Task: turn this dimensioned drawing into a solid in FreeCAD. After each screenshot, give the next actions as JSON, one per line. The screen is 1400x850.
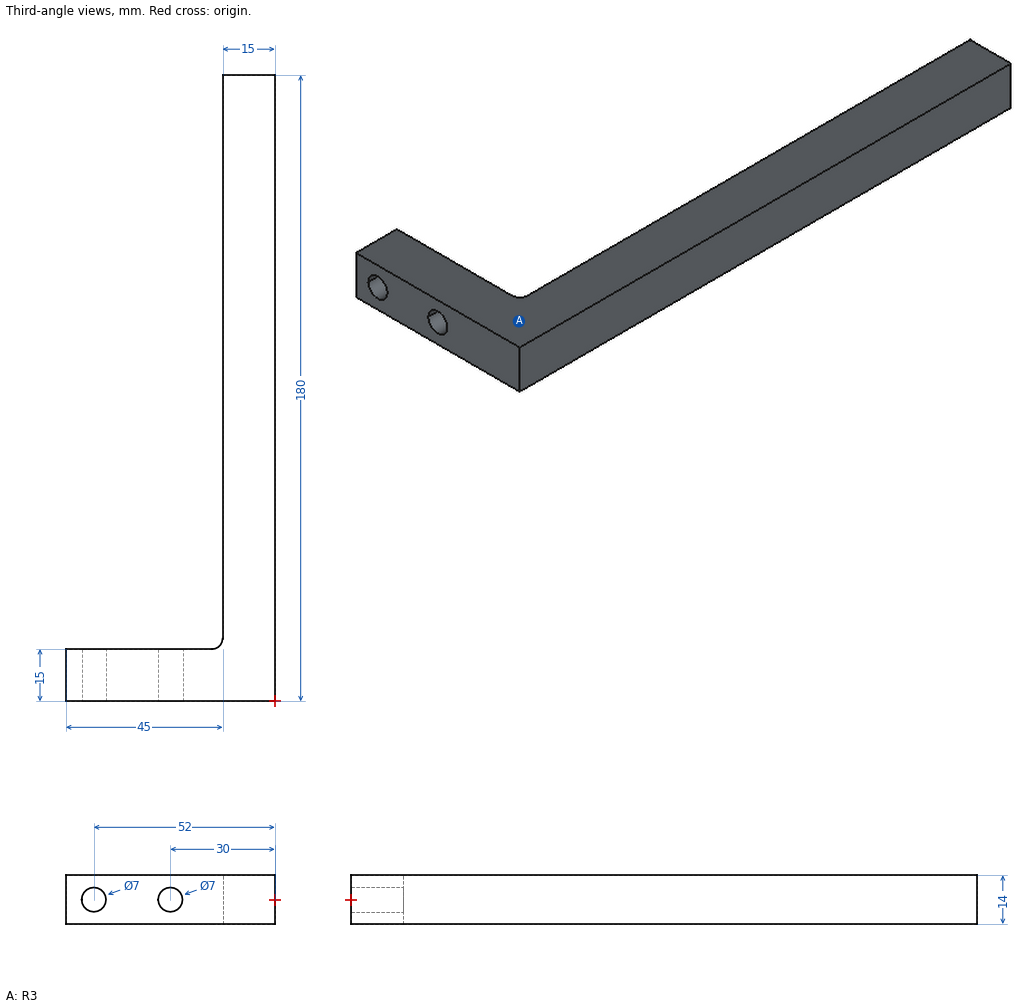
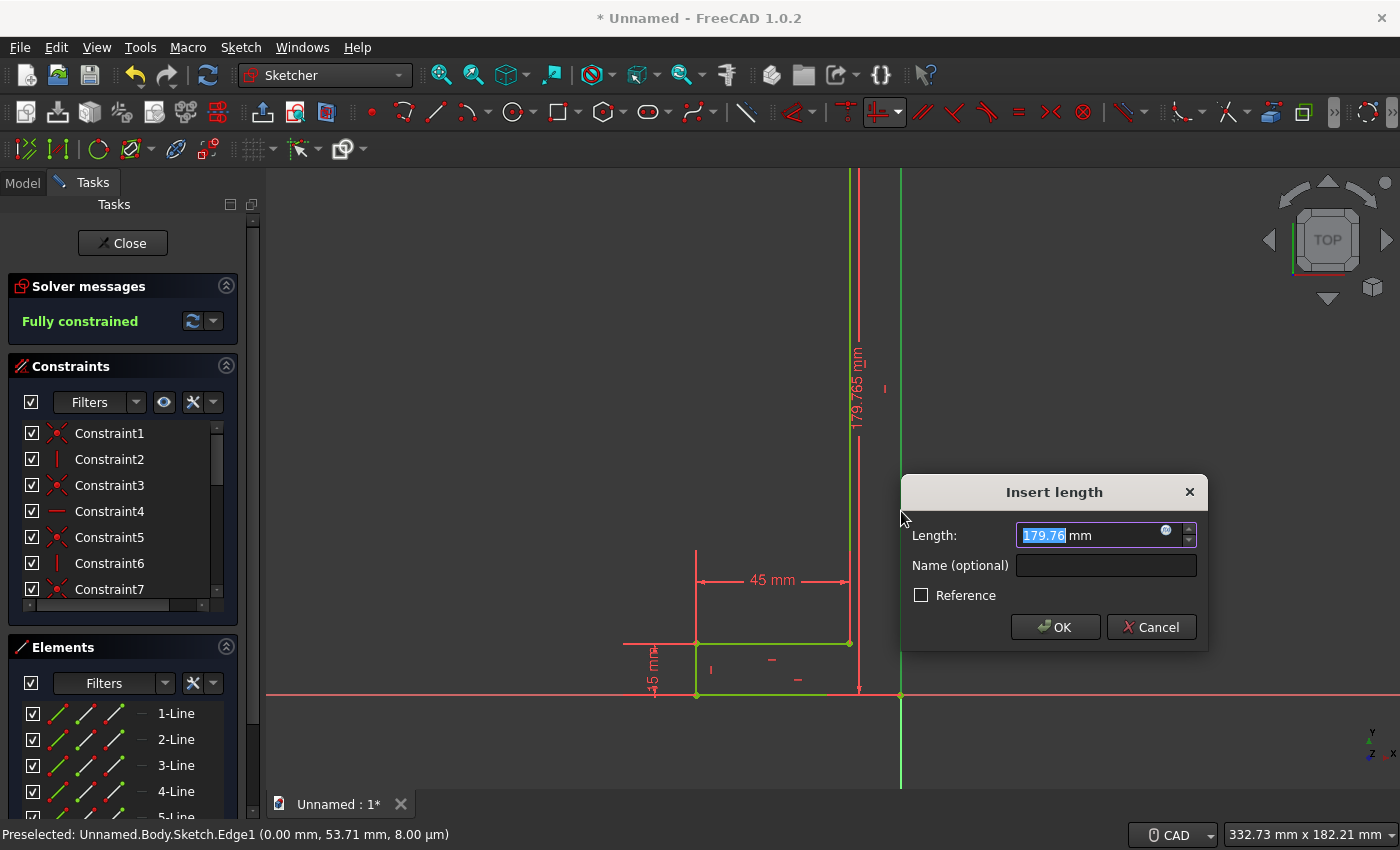
{"action": "type", "text": "180"}
{"action": "key", "text": "Return"}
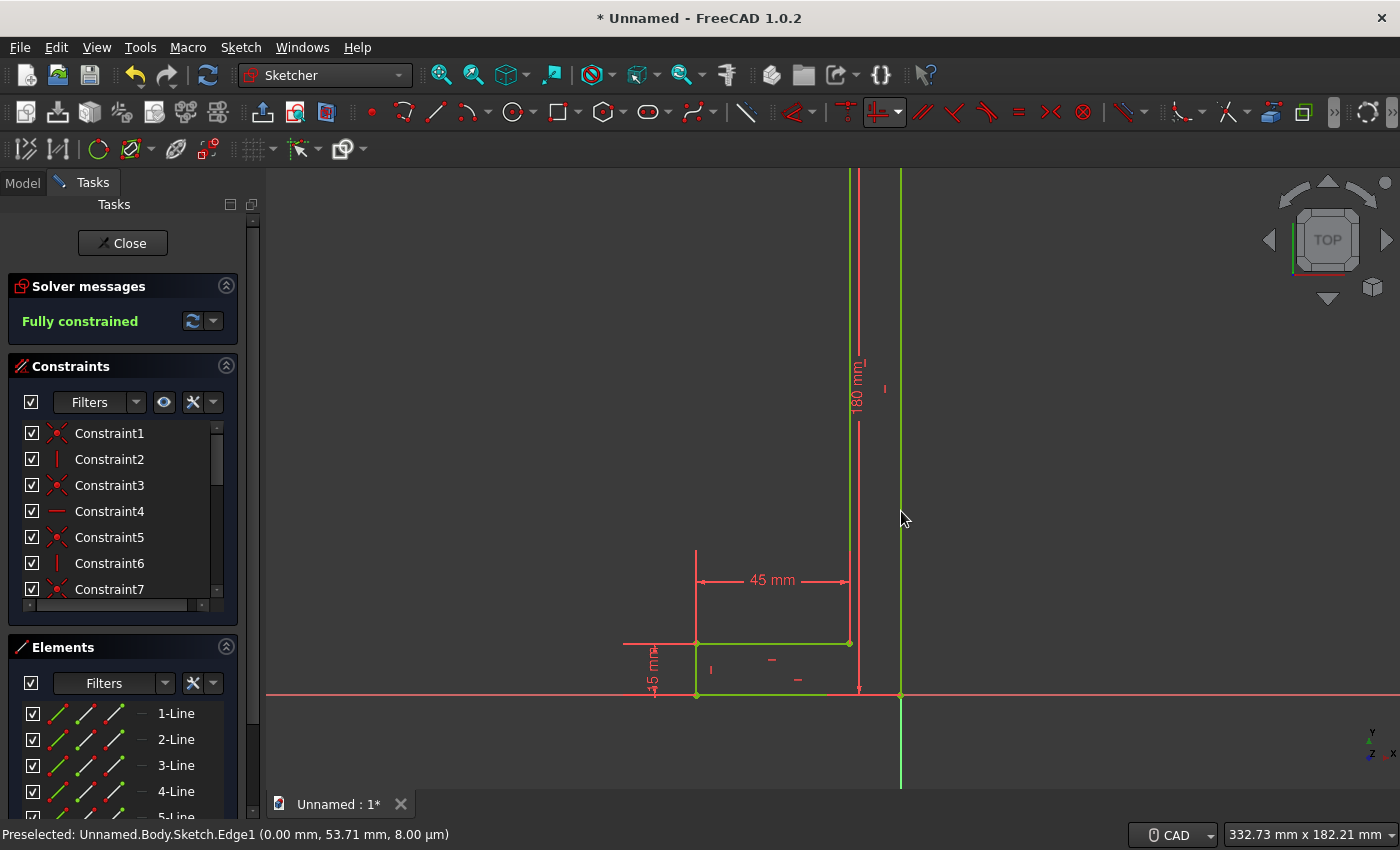
{"action": "left_click", "coordinate": [123, 243]}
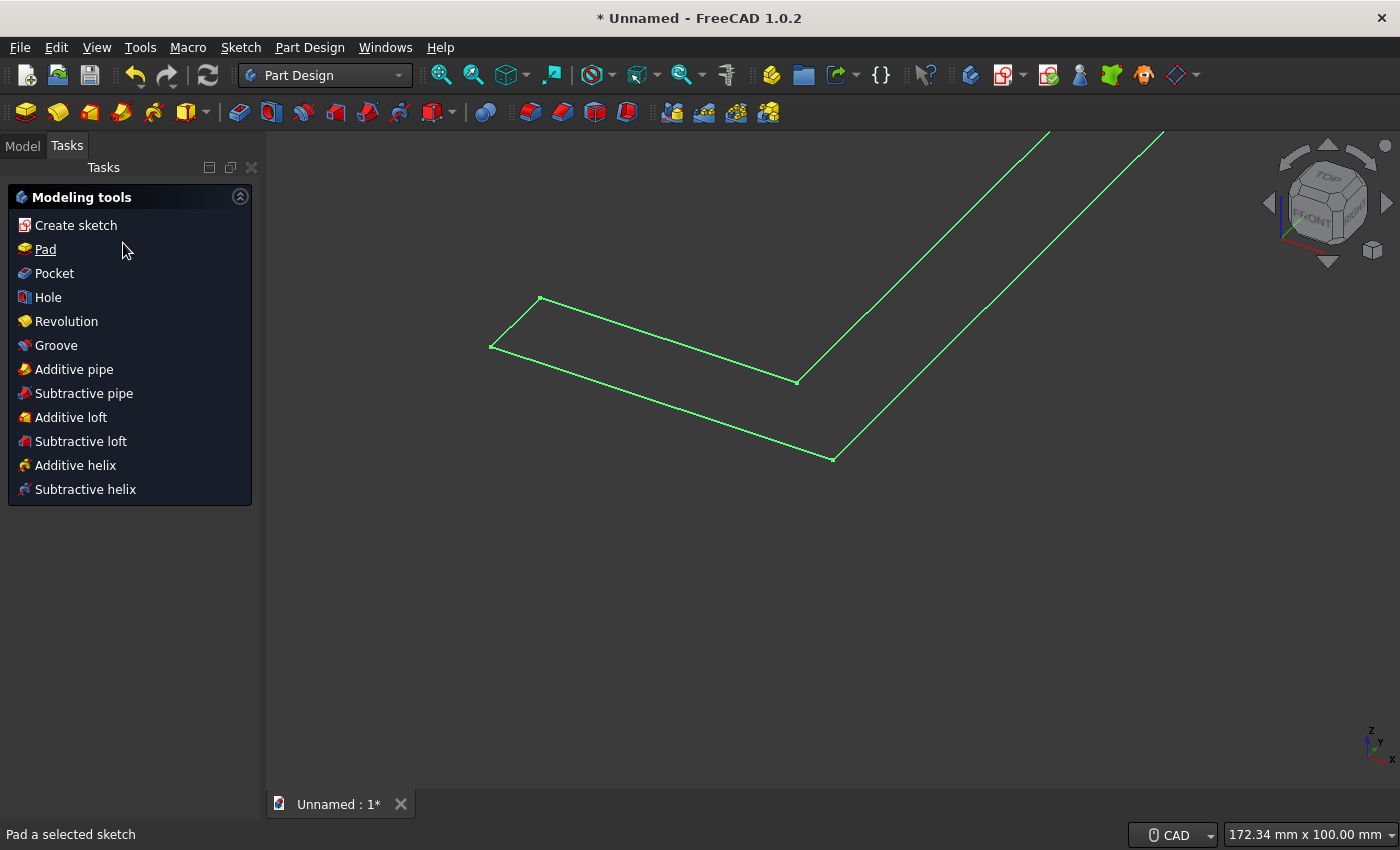
{"action": "left_click", "coordinate": [26, 112]}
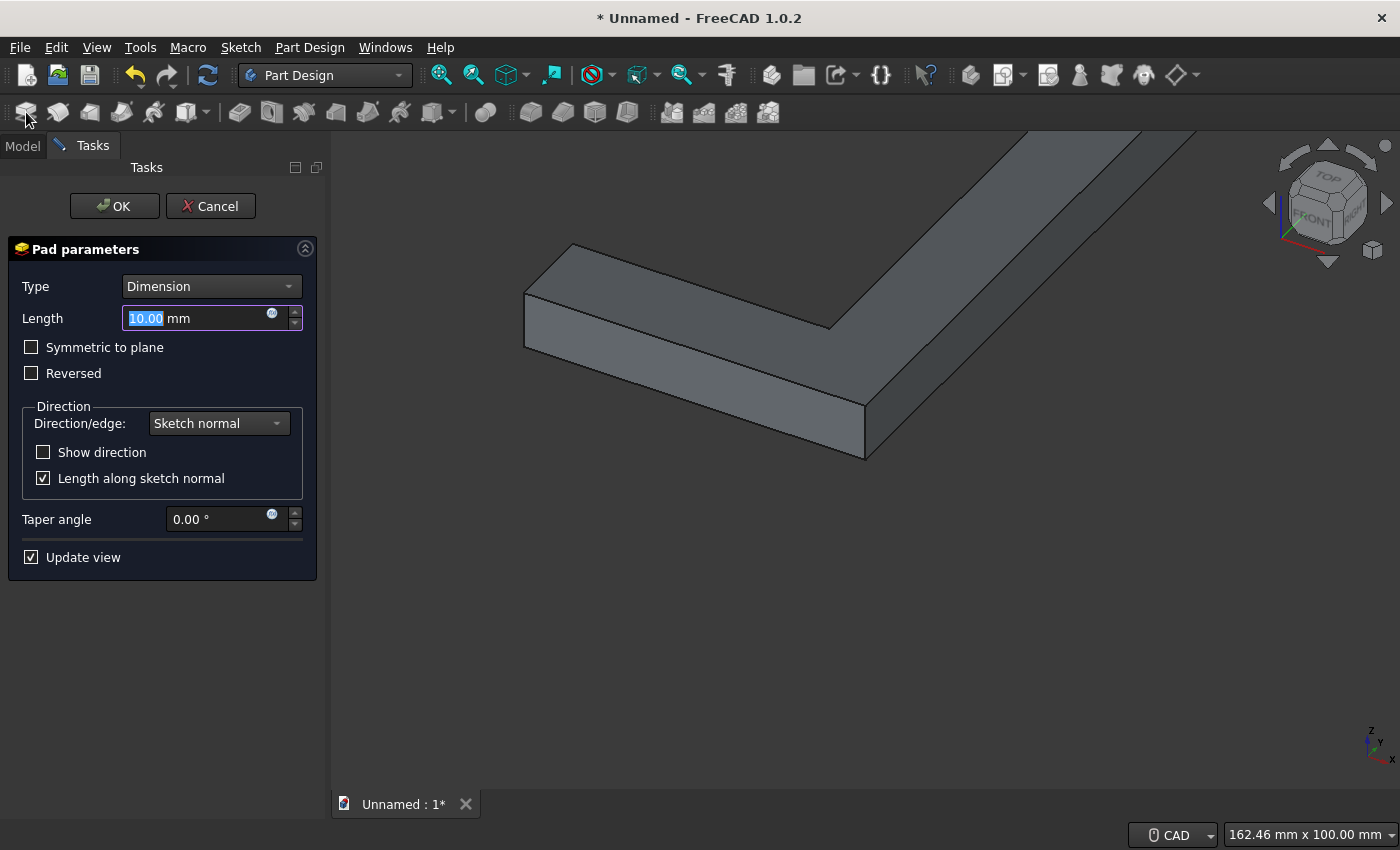
{"action": "type", "text": "14"}
{"action": "key", "text": "Tab"}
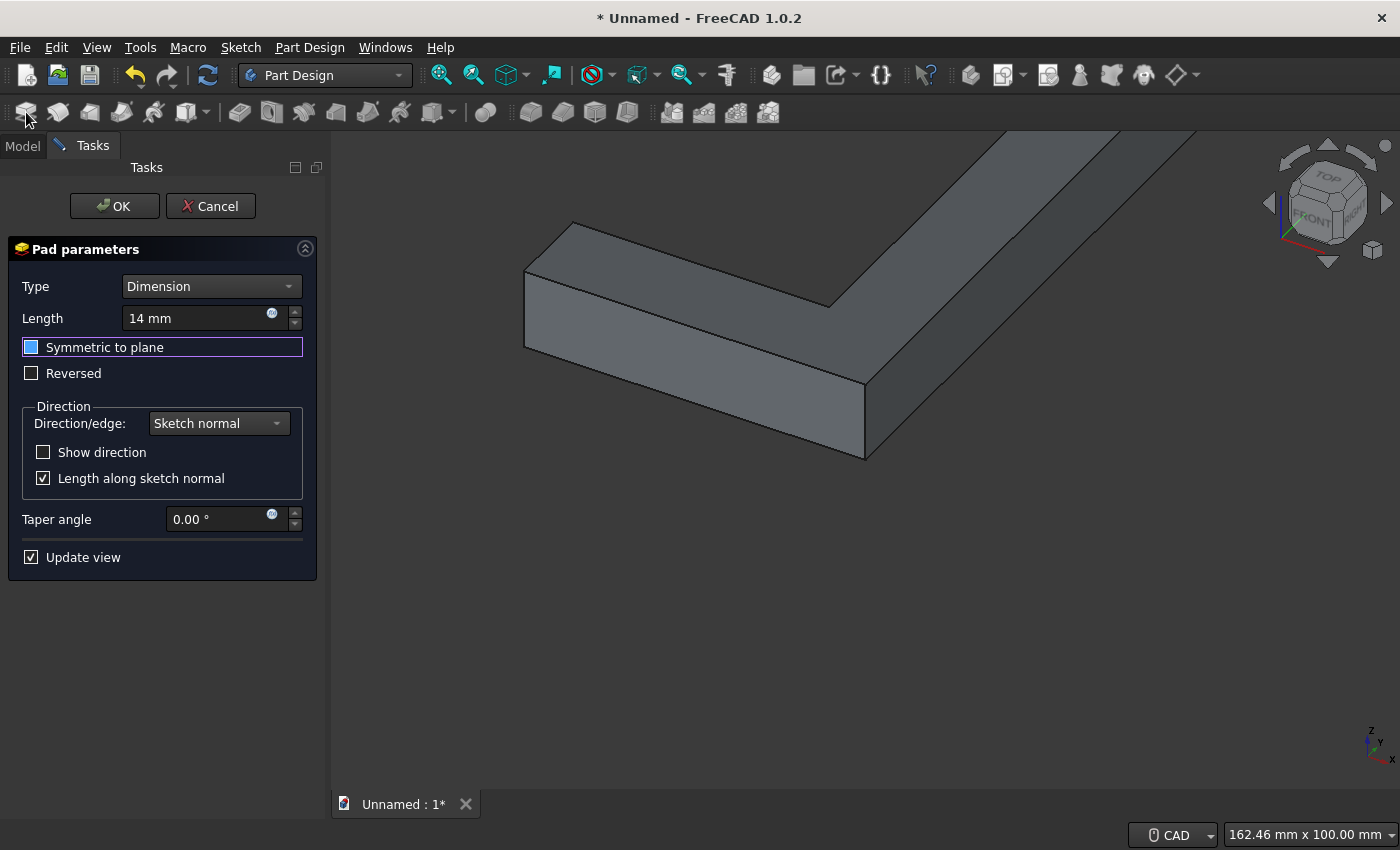
{"action": "left_click", "coordinate": [30, 347]}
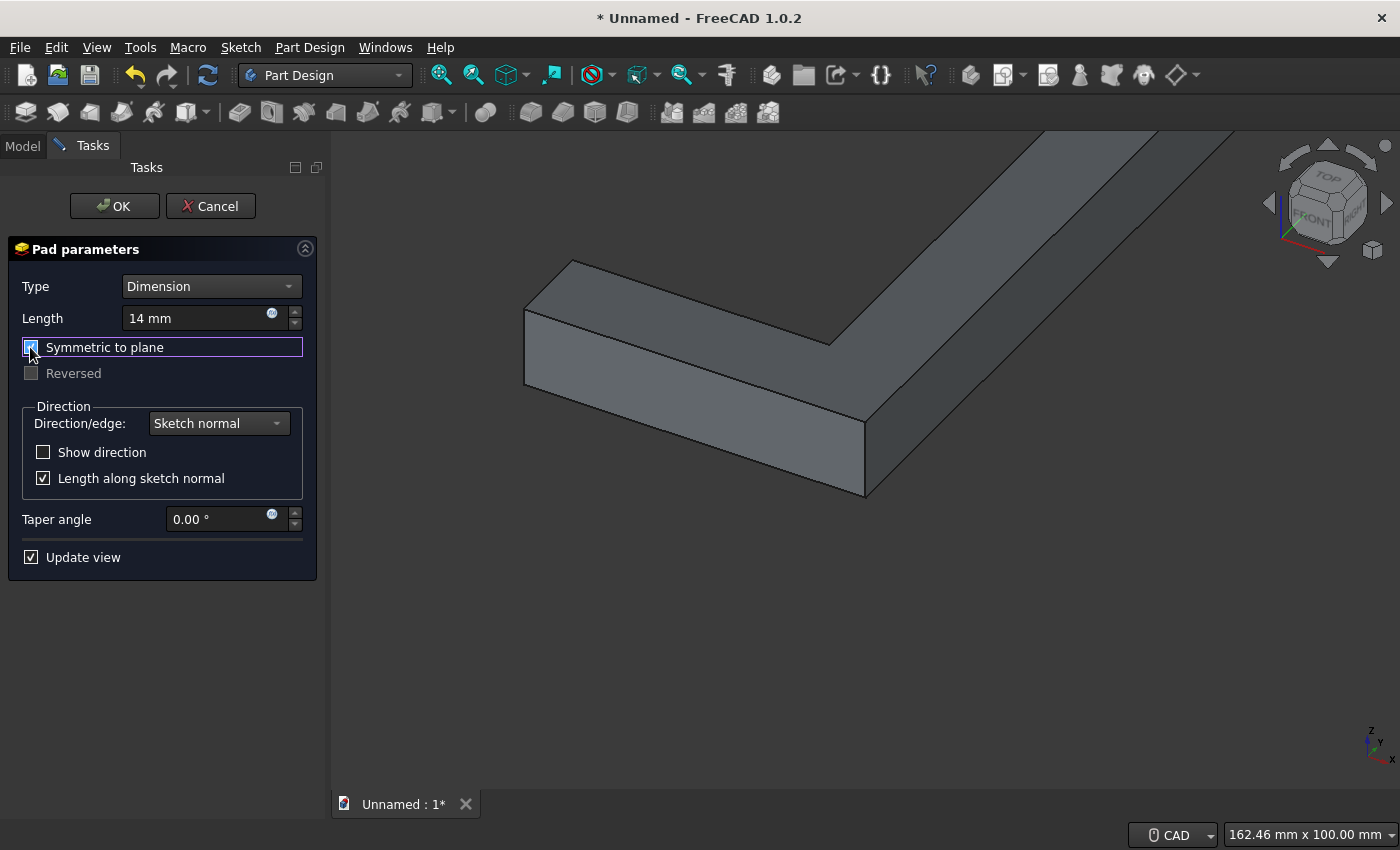
{"action": "left_click", "coordinate": [115, 206]}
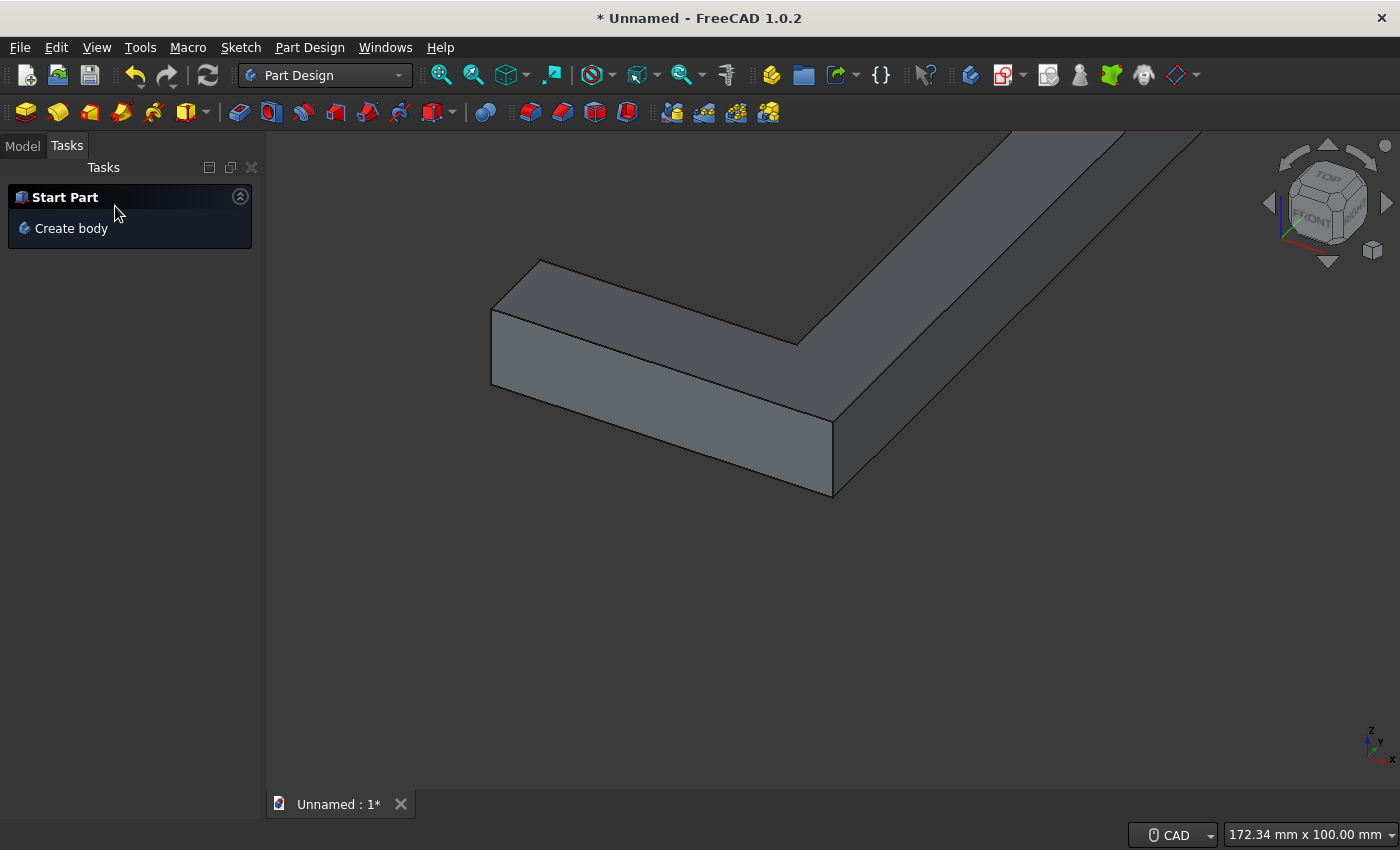
{"action": "key", "text": "v f"}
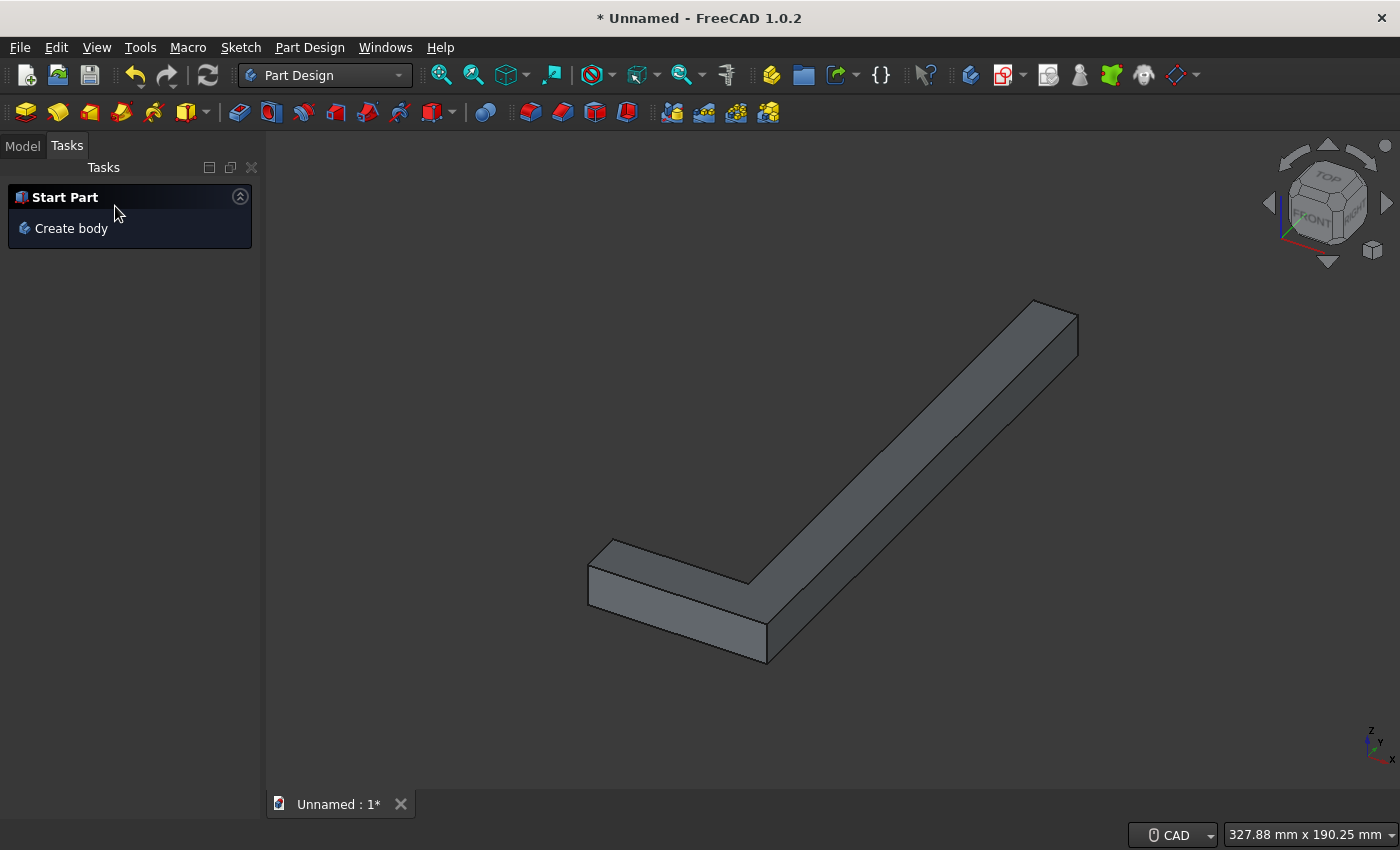
{"action": "key", "text": "0"}